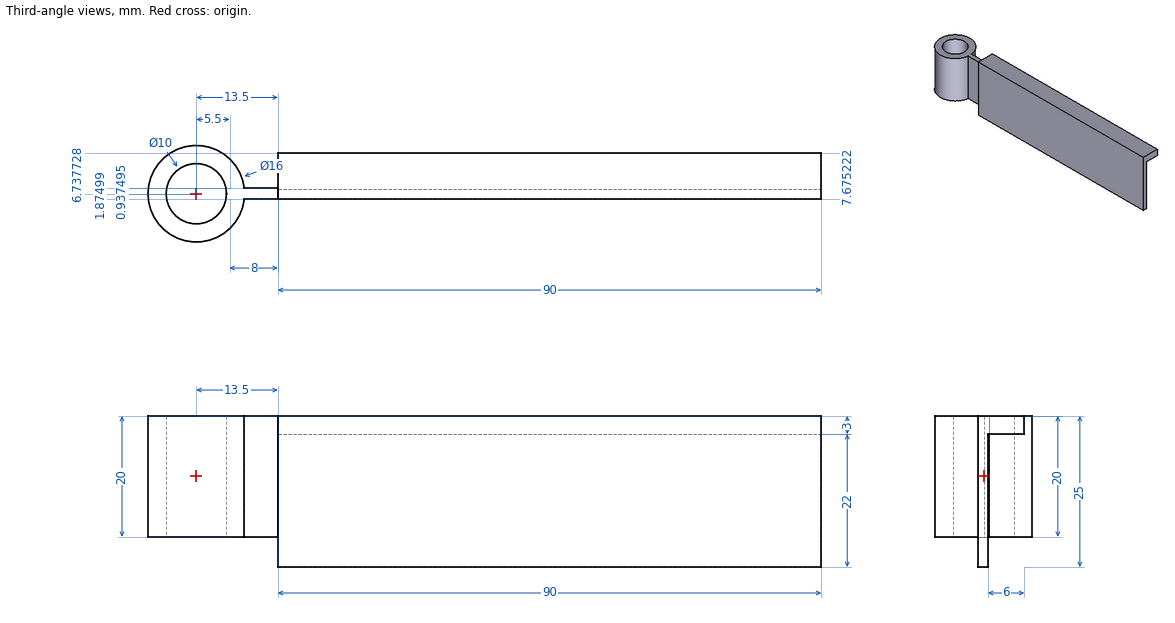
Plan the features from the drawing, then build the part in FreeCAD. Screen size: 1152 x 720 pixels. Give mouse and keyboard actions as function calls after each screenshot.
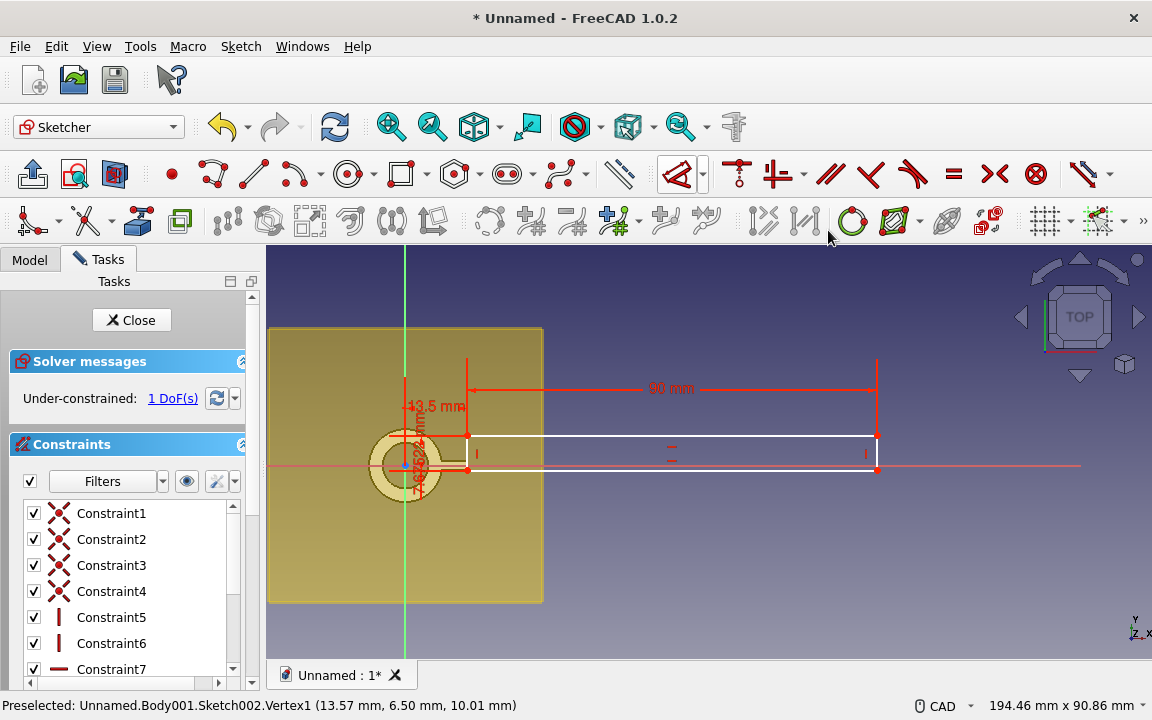
scroll(467, 436, up, 2)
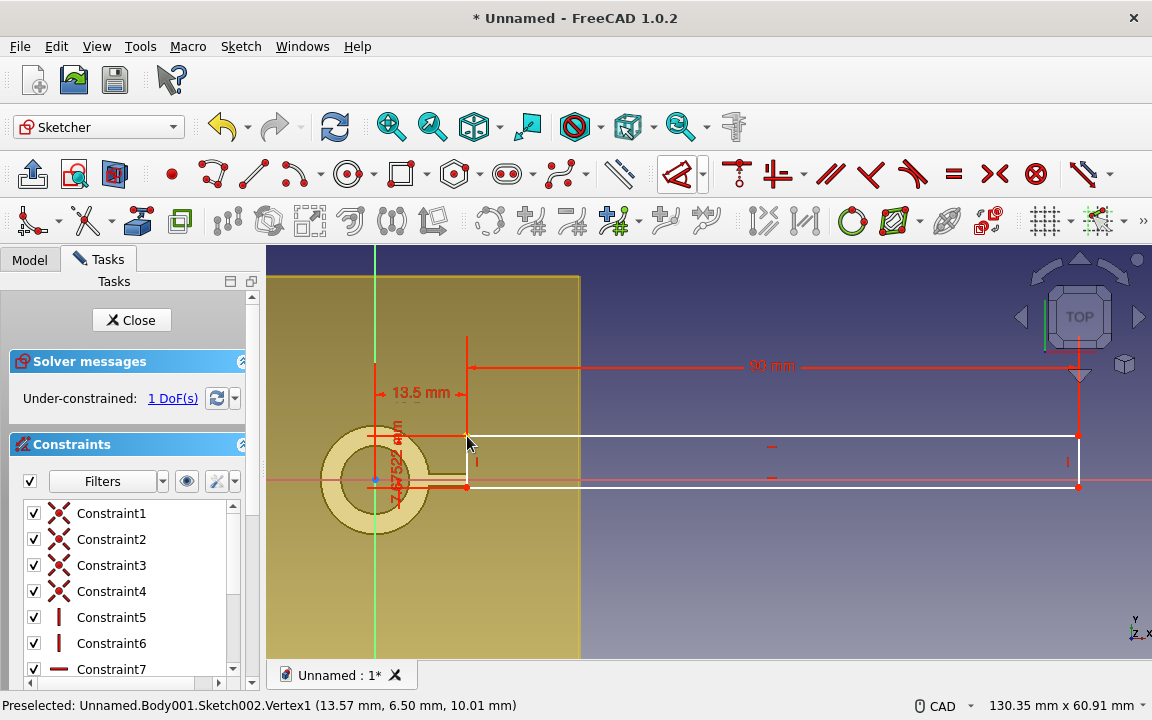
click(467, 436)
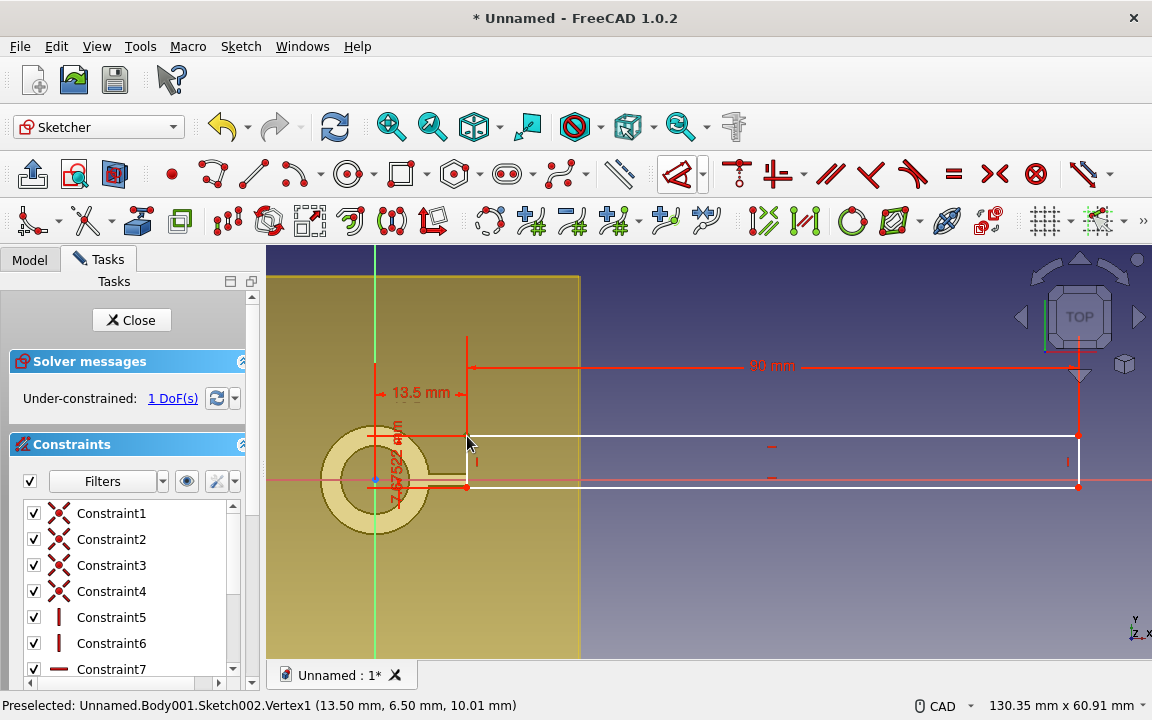
click(702, 174)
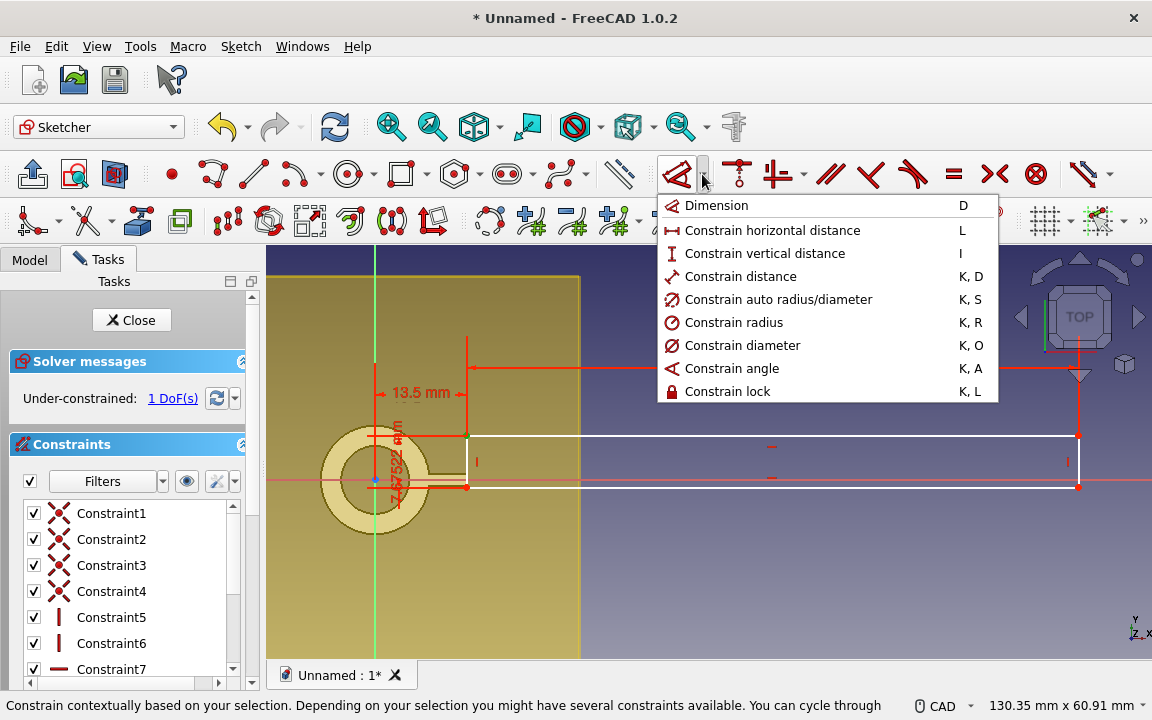
click(828, 254)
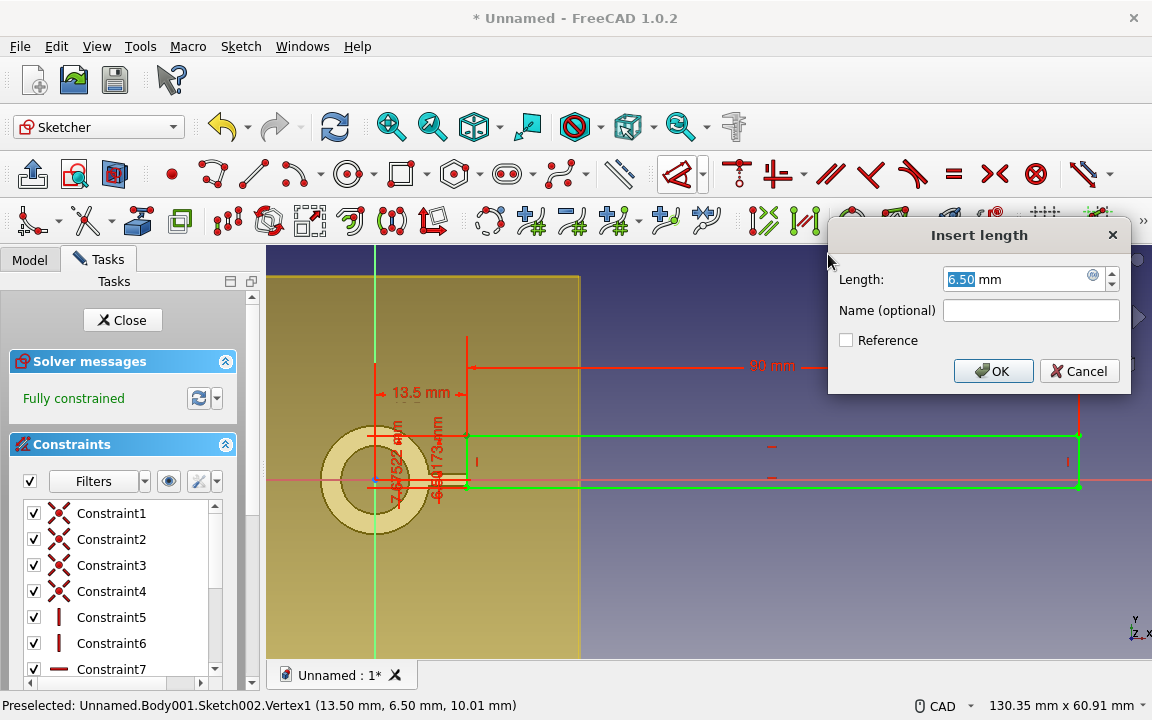
text(6.737728)
key(Return)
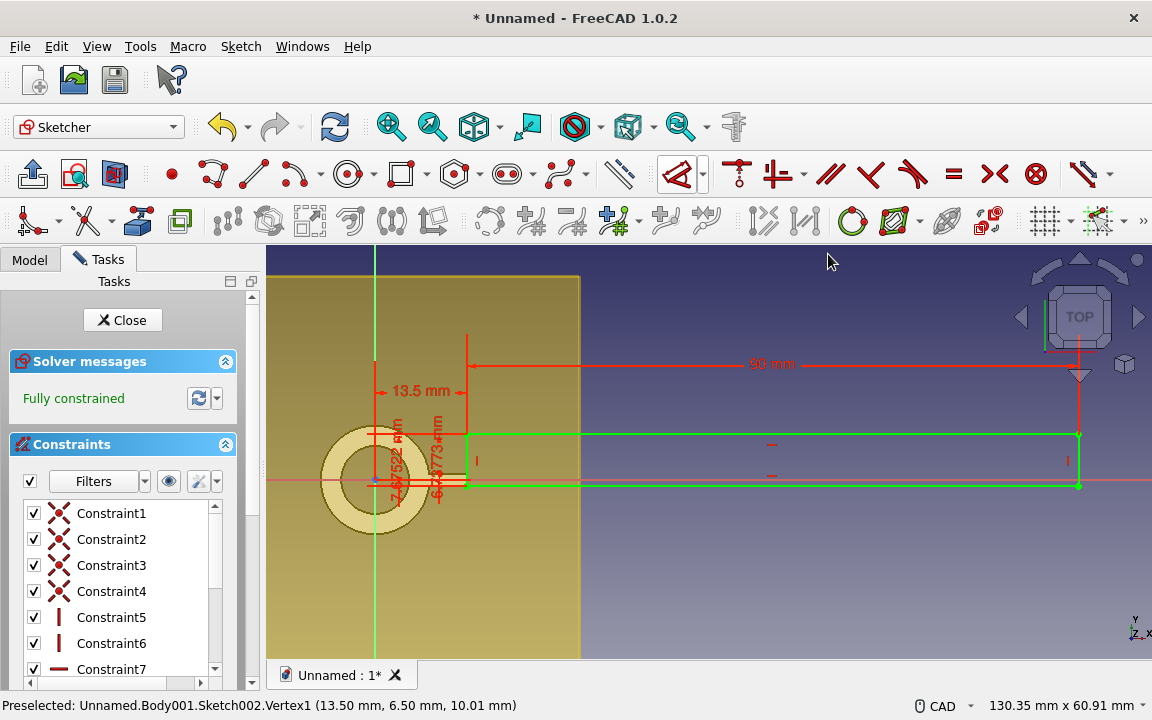
click(123, 320)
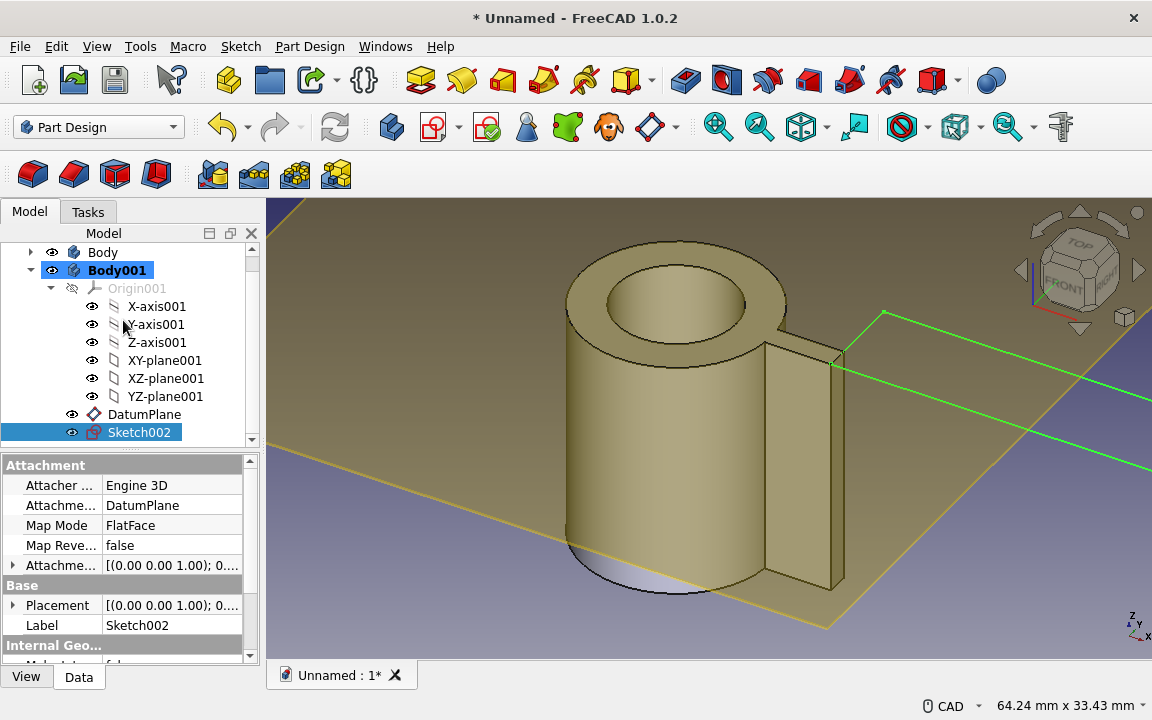
click(421, 80)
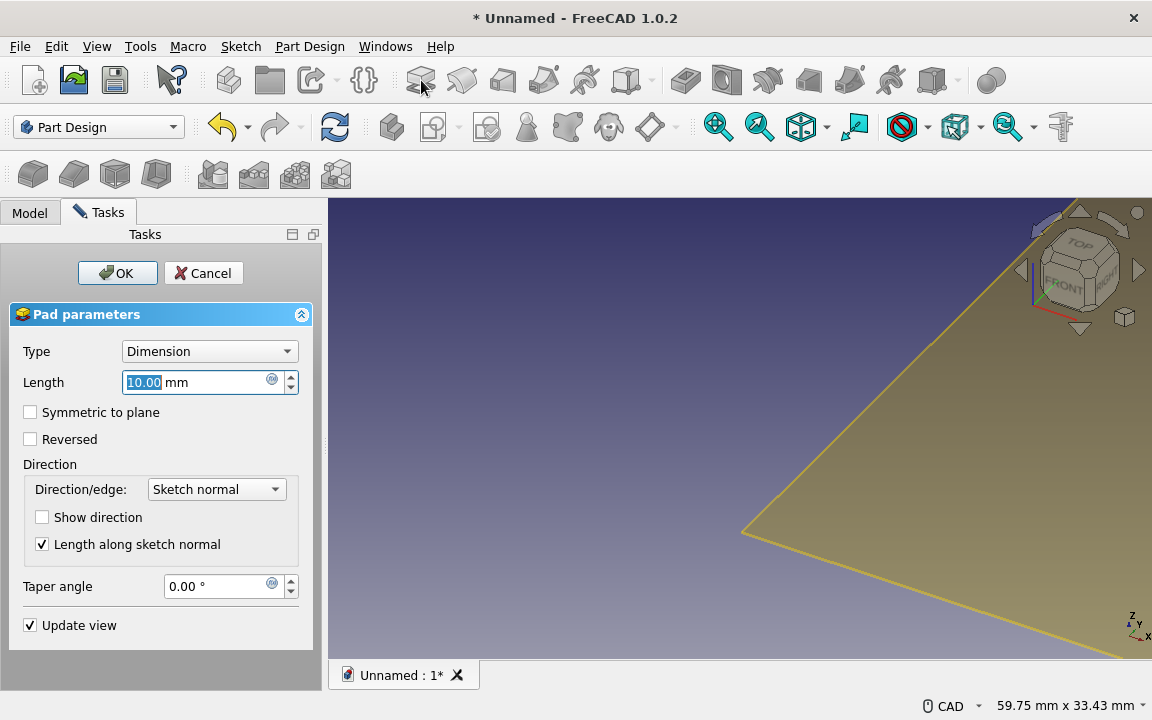
text(25)
key(Tab)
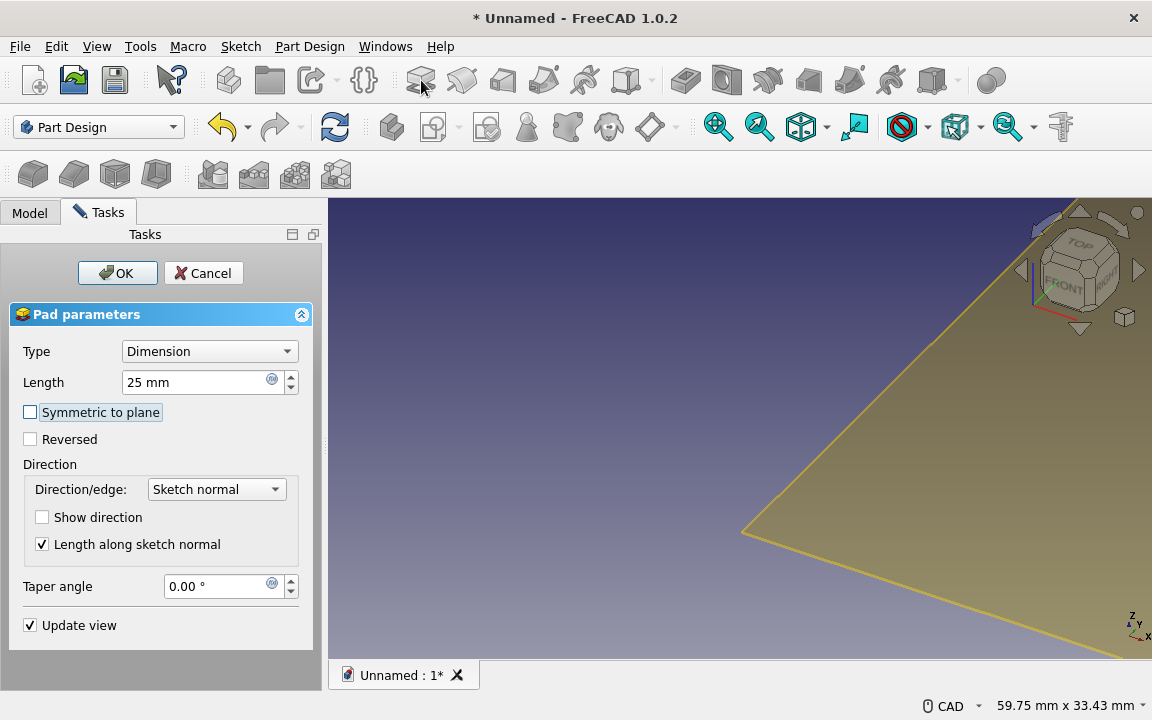
click(31, 439)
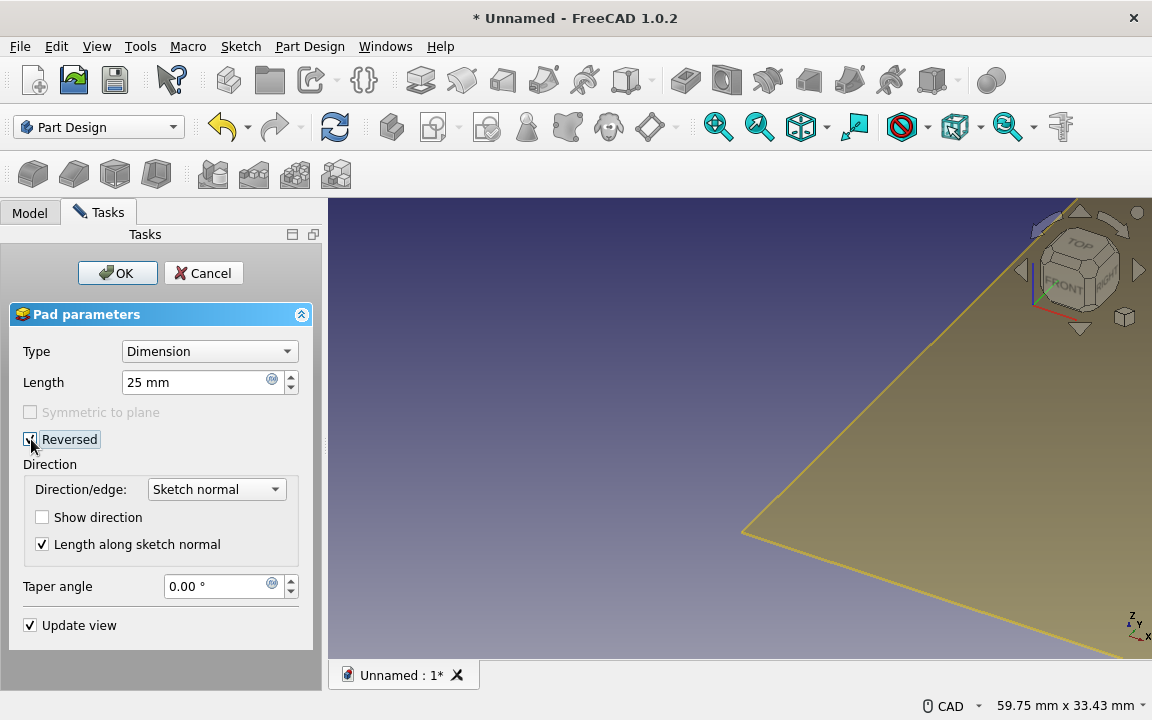
click(118, 273)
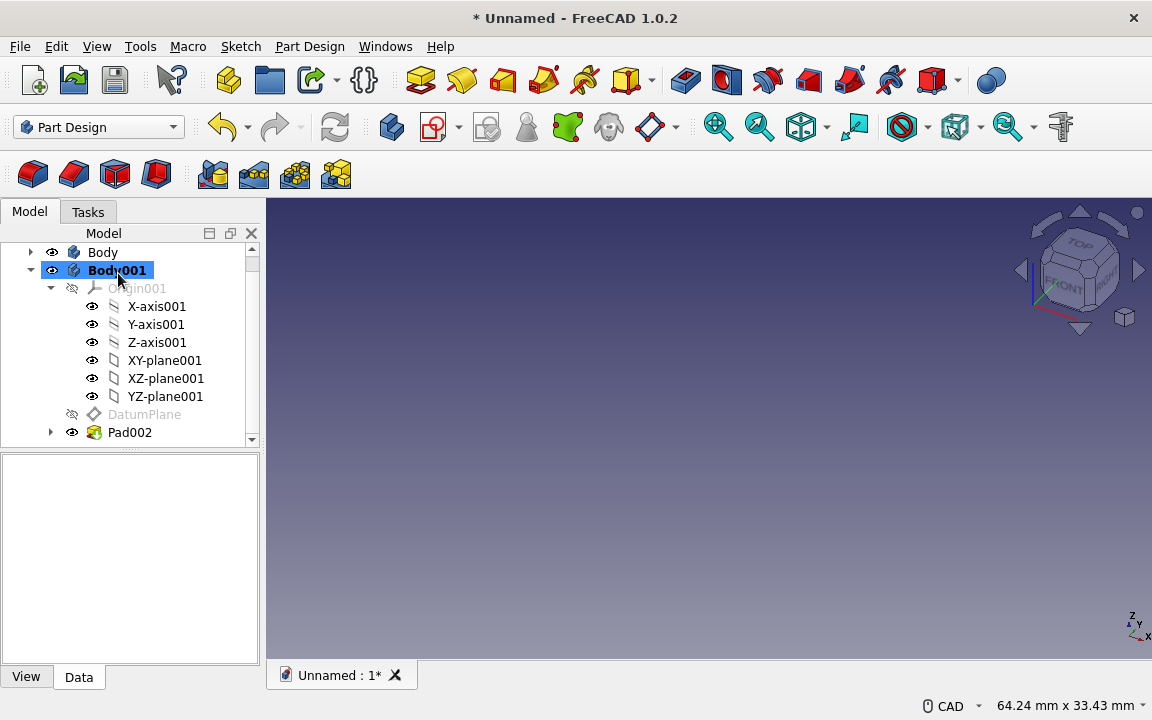
click(719, 128)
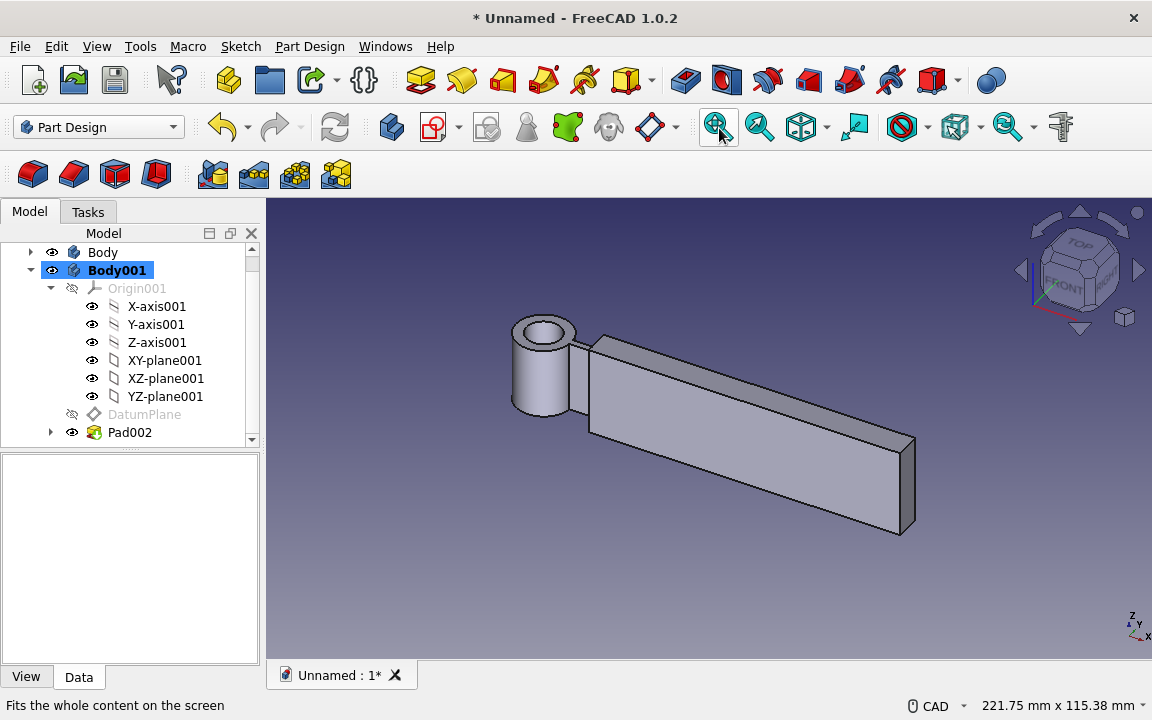
key(4)